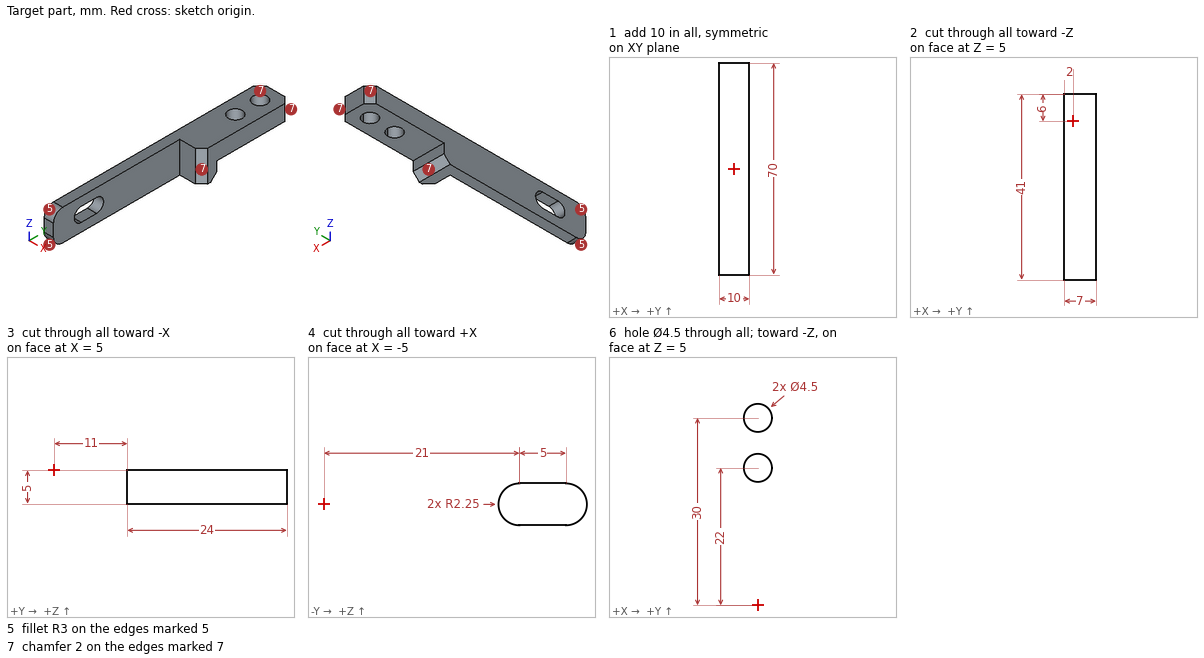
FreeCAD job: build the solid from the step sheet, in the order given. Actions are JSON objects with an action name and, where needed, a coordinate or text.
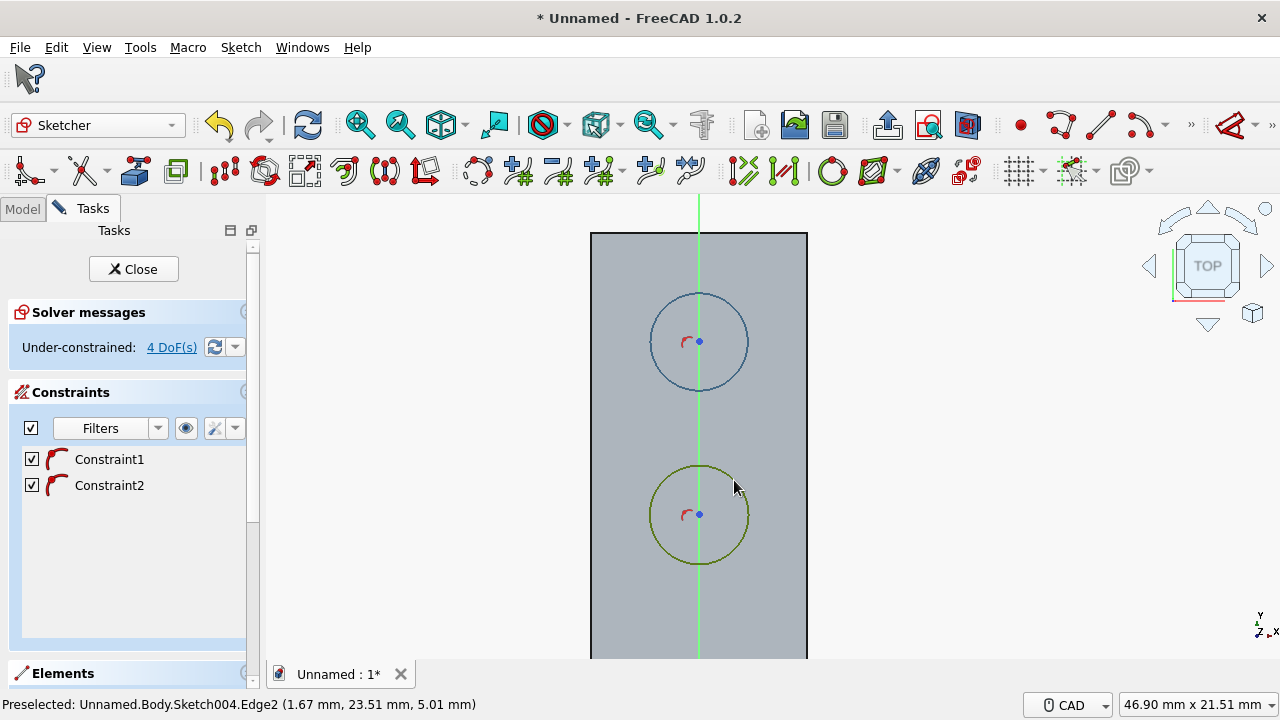
{"action": "key", "text": "e"}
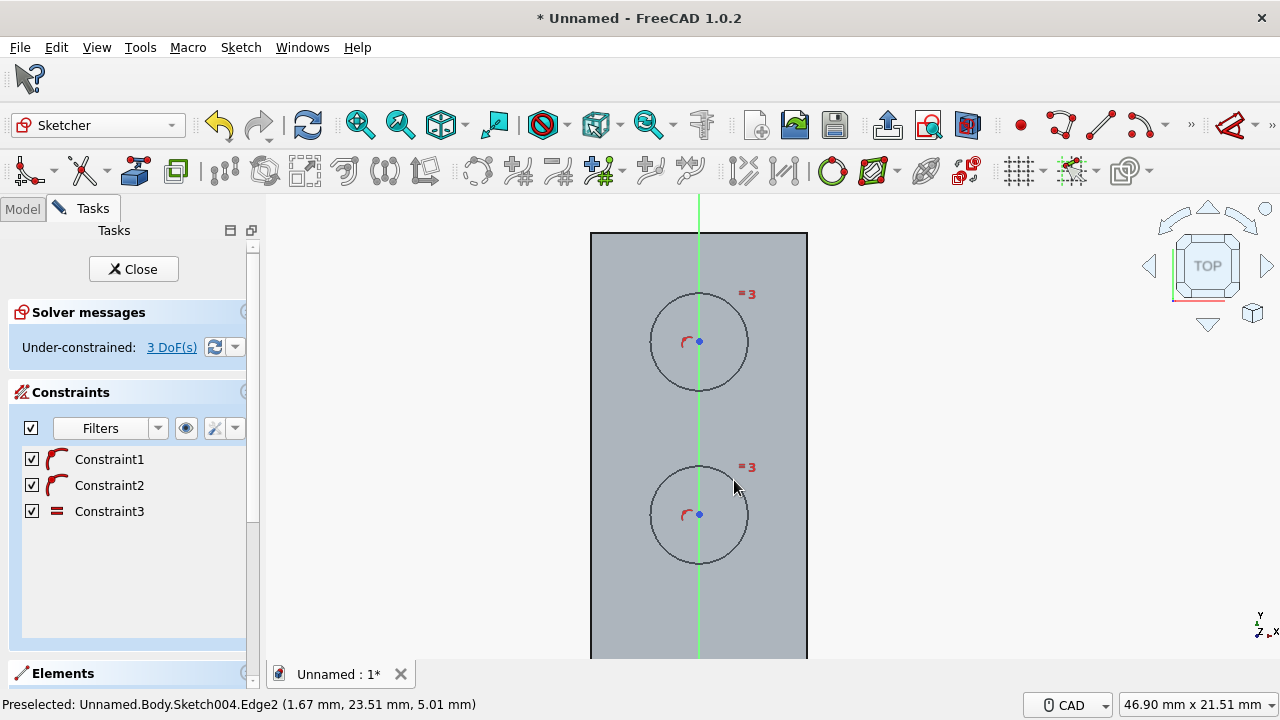
{"action": "key", "text": "d"}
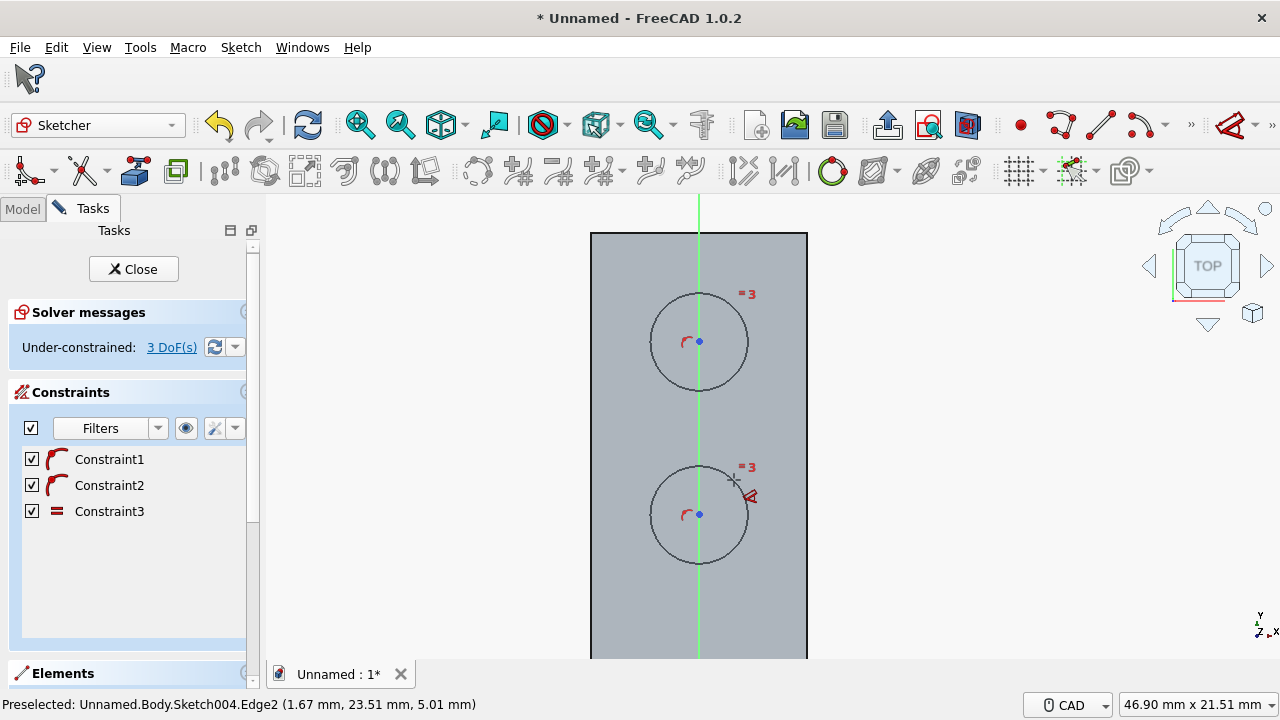
{"action": "left_click", "coordinate": [733, 307]}
{"action": "left_click", "coordinate": [755, 284]}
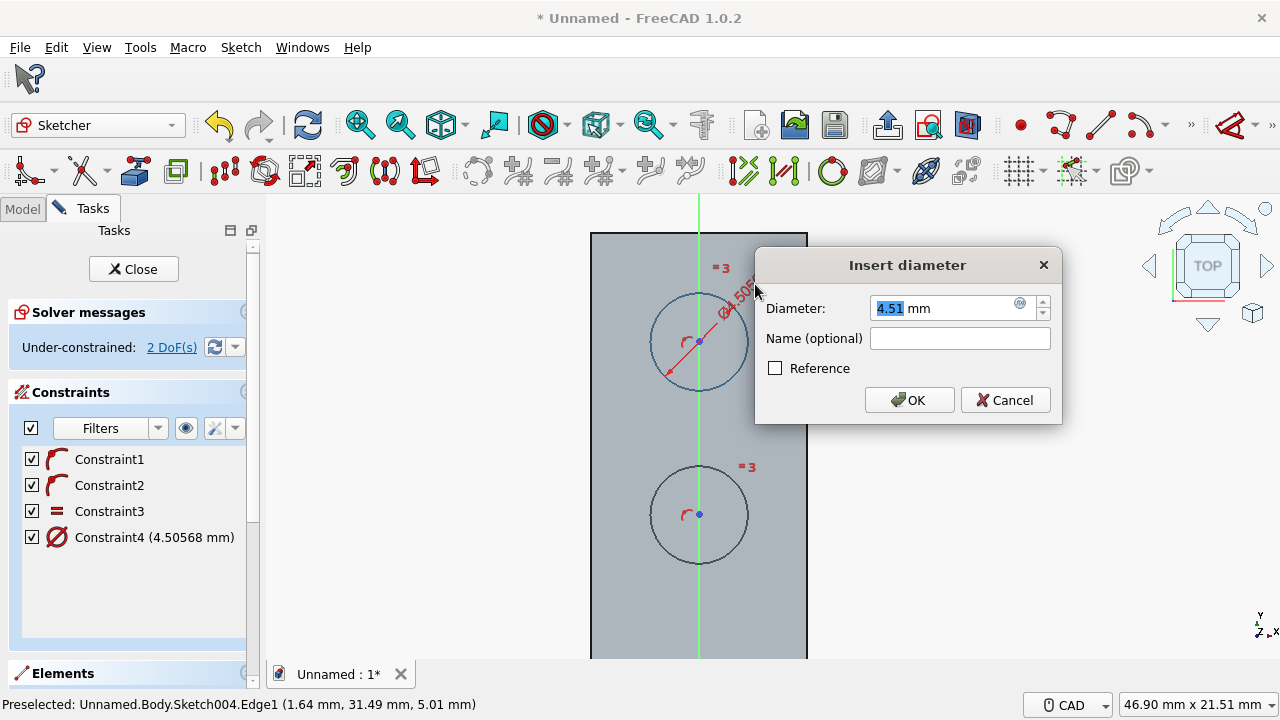
{"action": "type", "text": "4.5"}
{"action": "key", "text": "Return"}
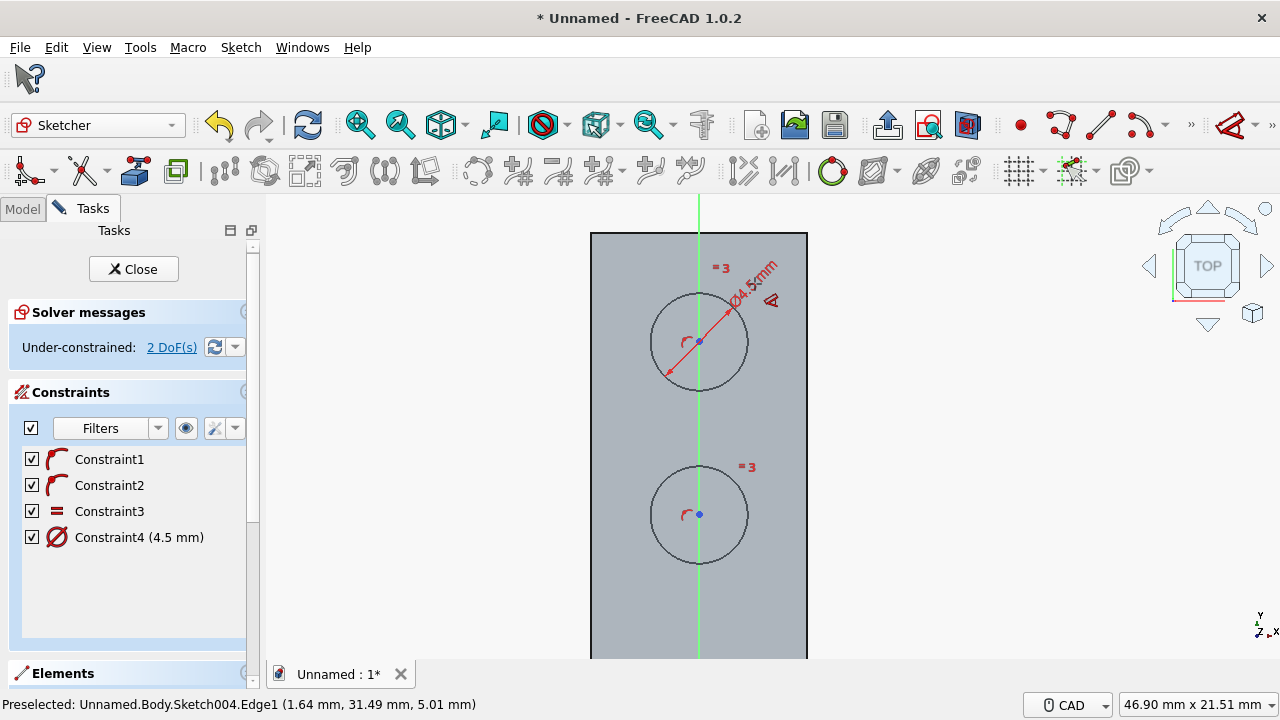
{"action": "left_click", "coordinate": [699, 342]}
{"action": "left_click", "coordinate": [733, 420]}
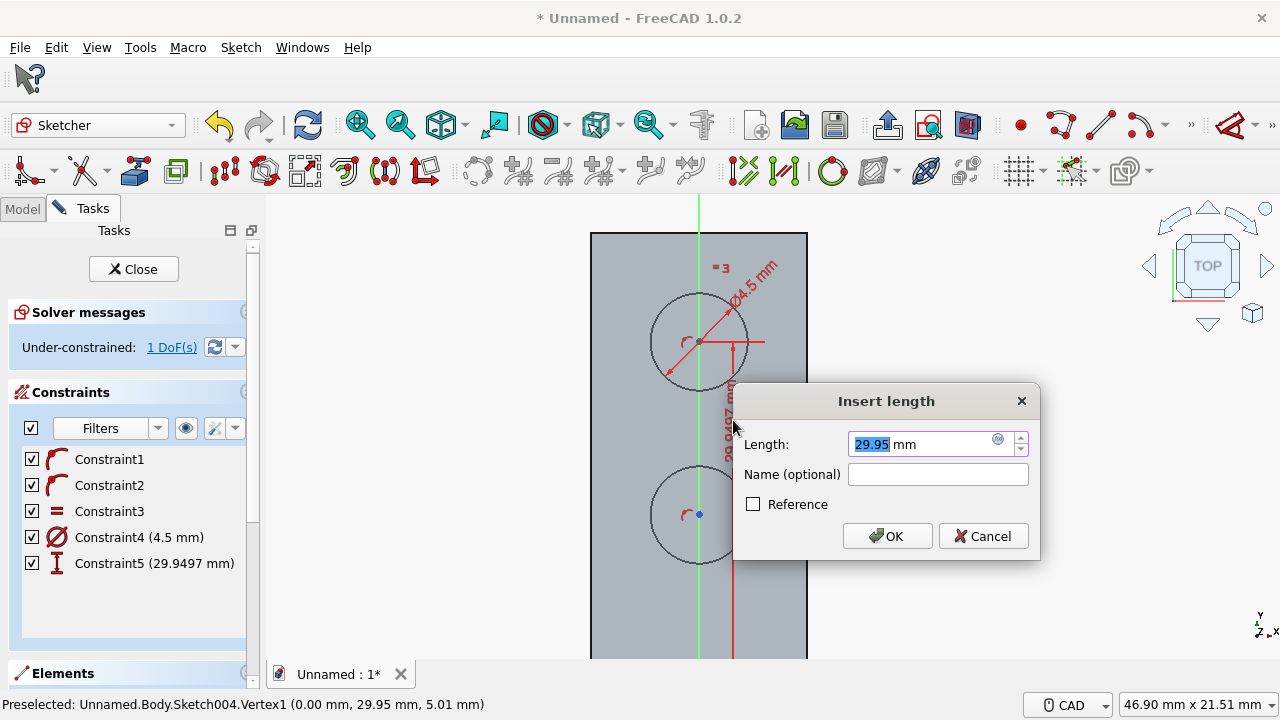
{"action": "type", "text": "30"}
{"action": "key", "text": "Return"}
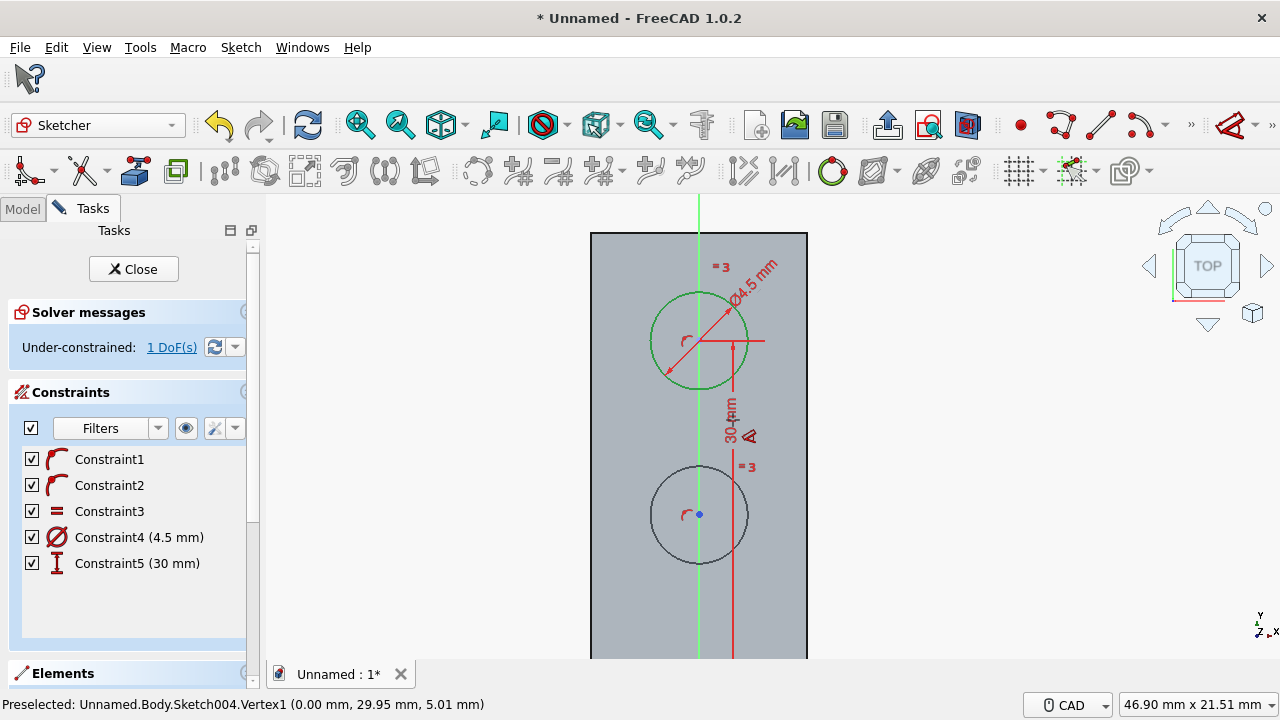
{"action": "left_click", "coordinate": [699, 515]}
{"action": "left_click", "coordinate": [733, 573]}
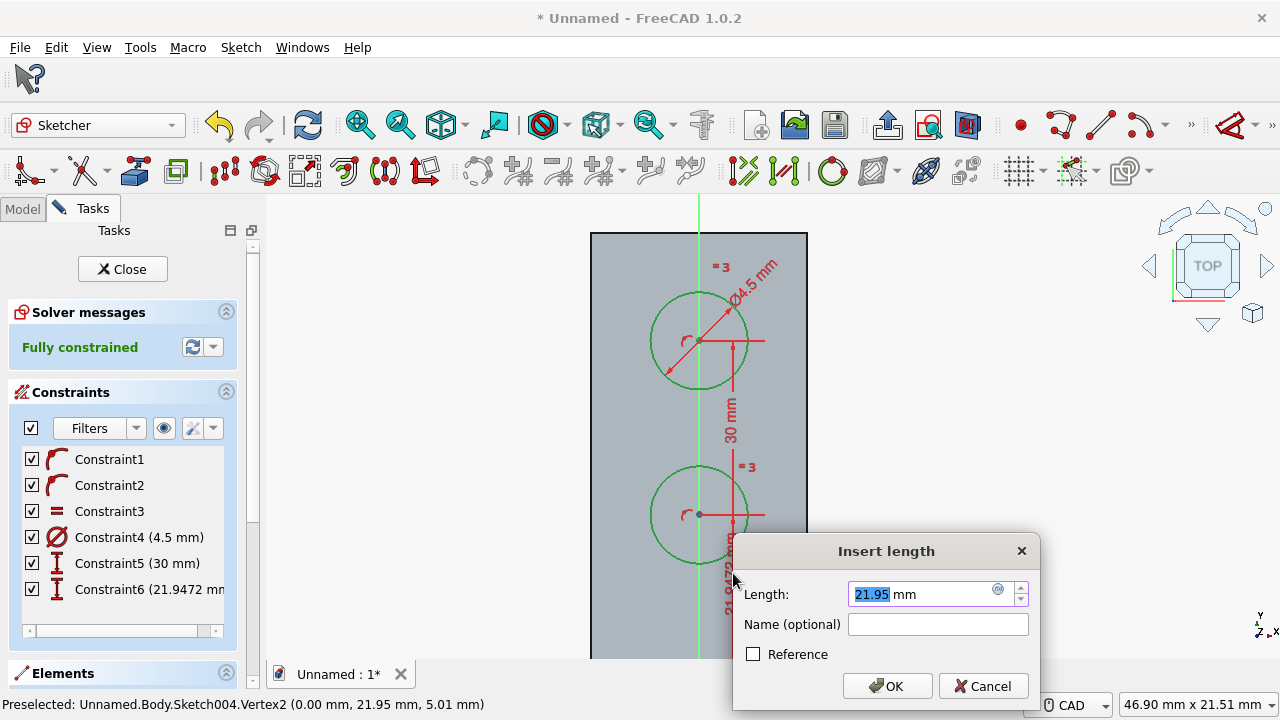
{"action": "type", "text": "22"}
{"action": "key", "text": "Return"}
{"action": "key", "text": "Escape"}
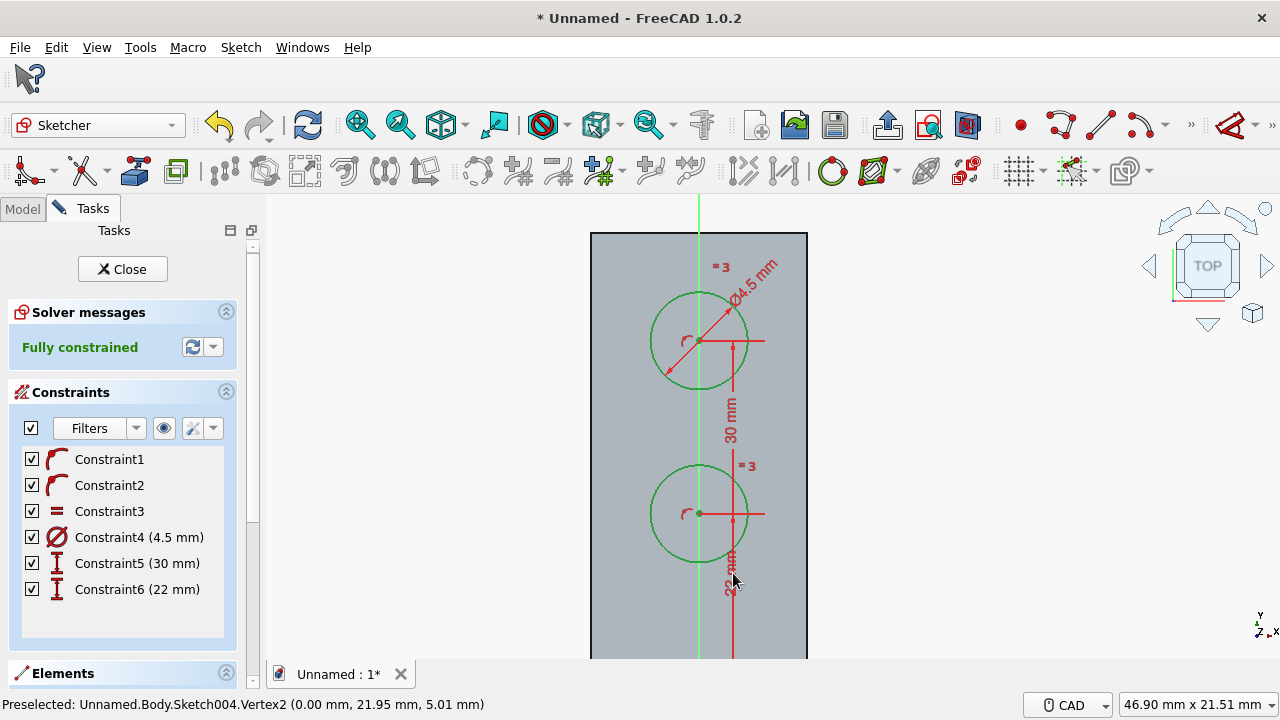
{"action": "left_click", "coordinate": [123, 269]}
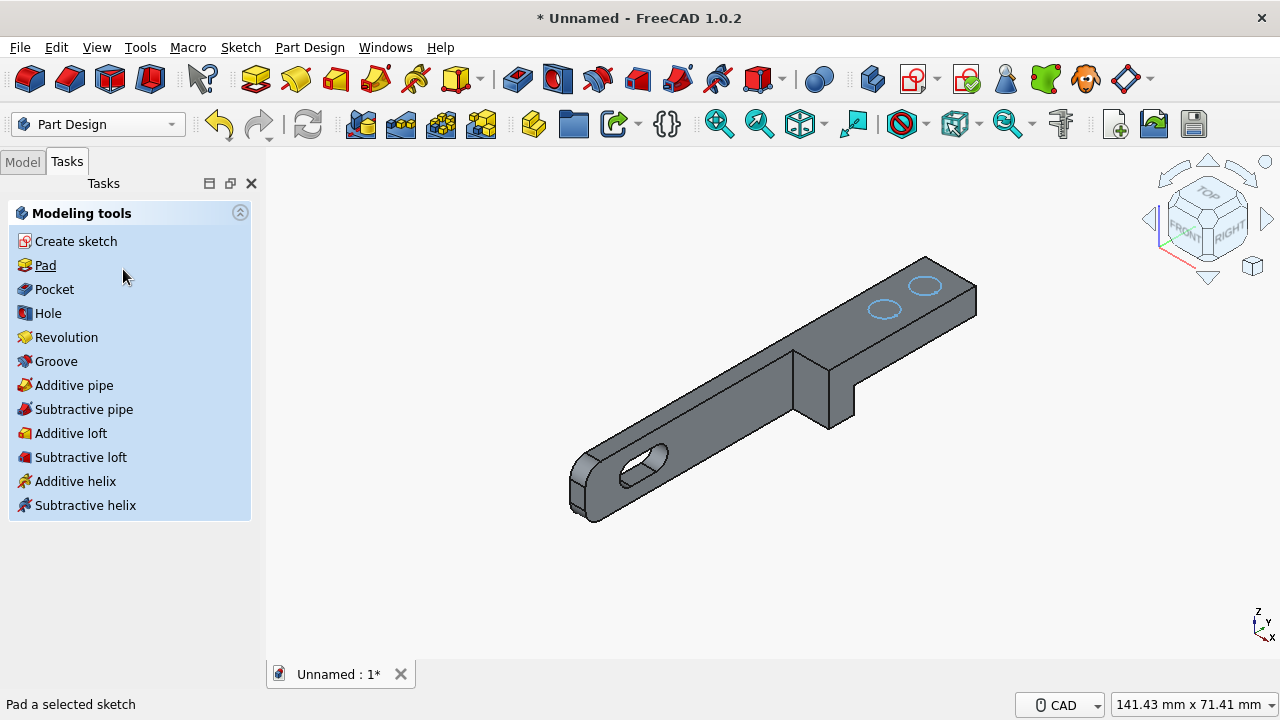
{"action": "left_click", "coordinate": [558, 80]}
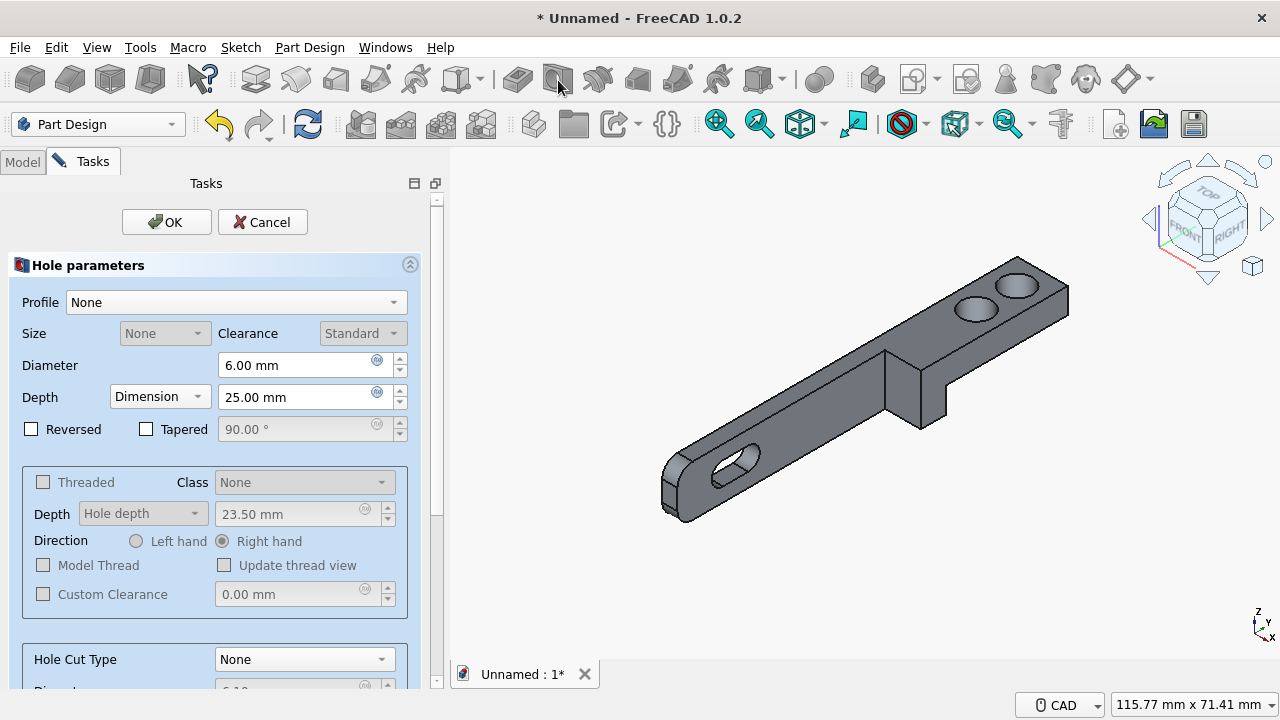
{"action": "triple_click", "coordinate": [305, 365]}